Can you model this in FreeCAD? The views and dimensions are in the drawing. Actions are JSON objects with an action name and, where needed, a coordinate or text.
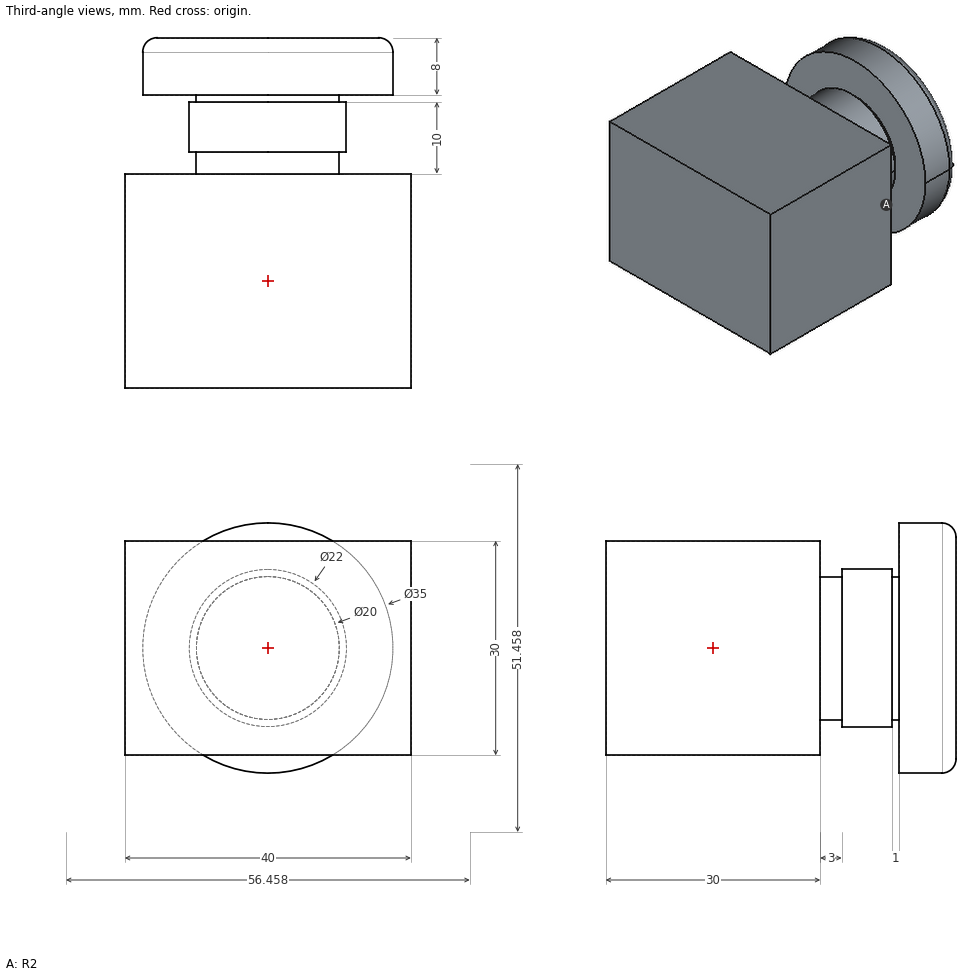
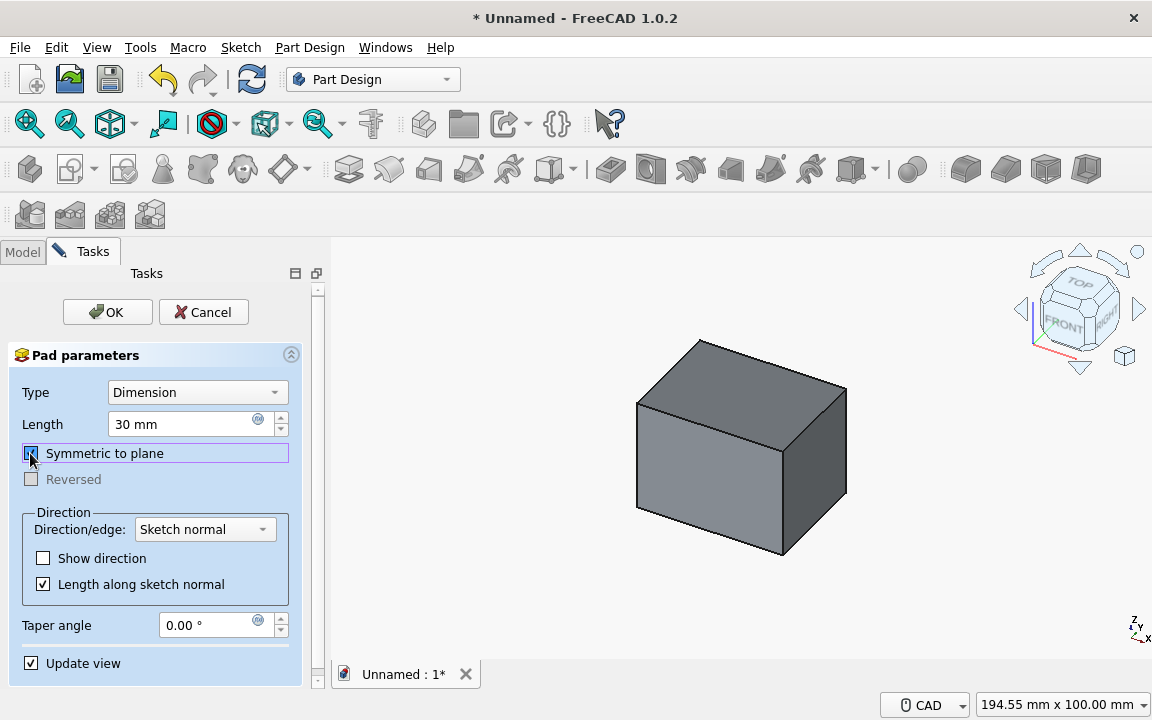
{"action": "left_click", "coordinate": [108, 312]}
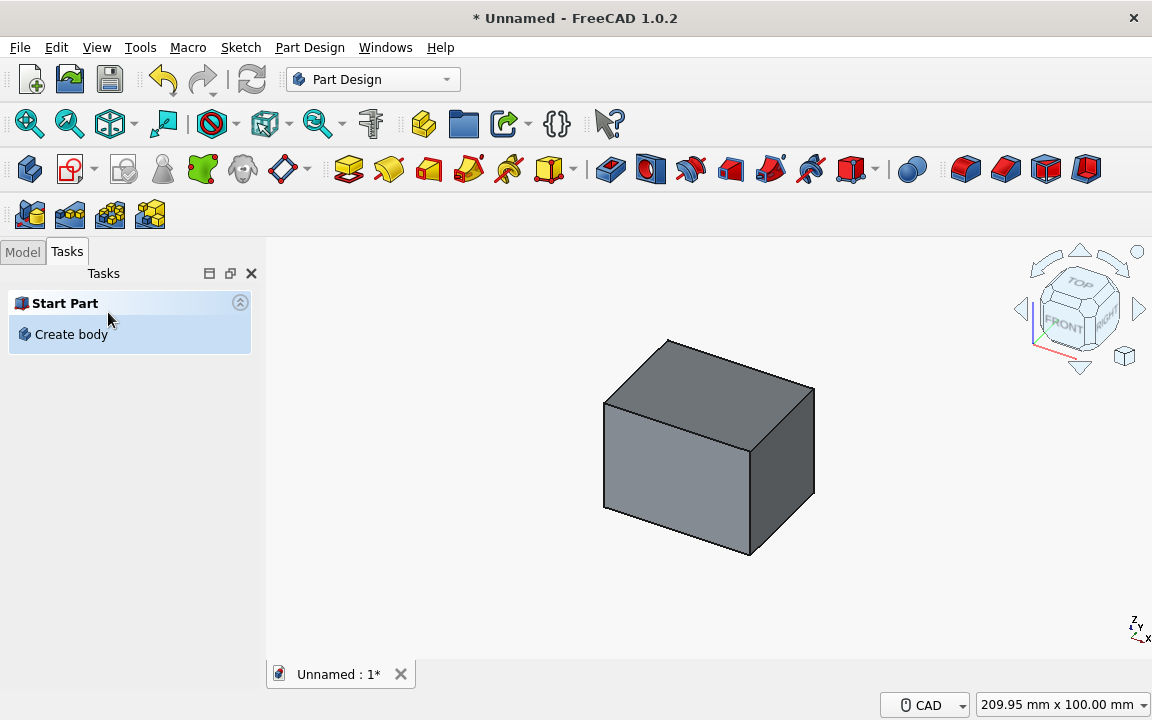
{"action": "key", "text": "4"}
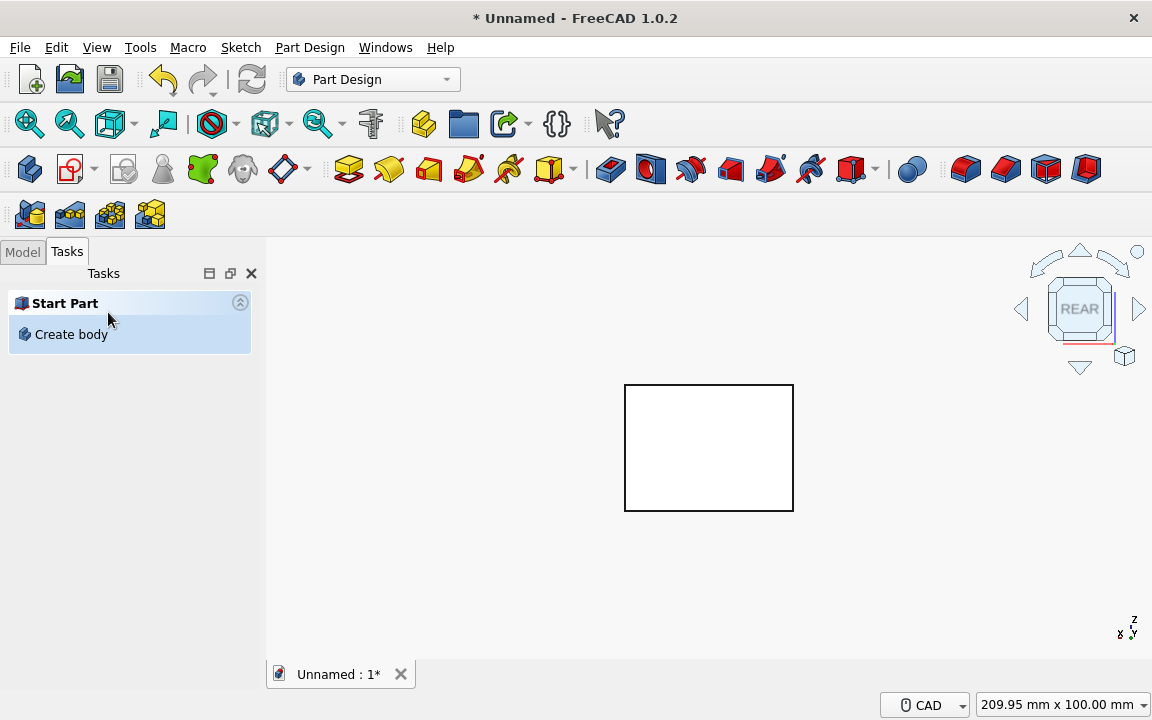
{"action": "left_click", "coordinate": [30, 124]}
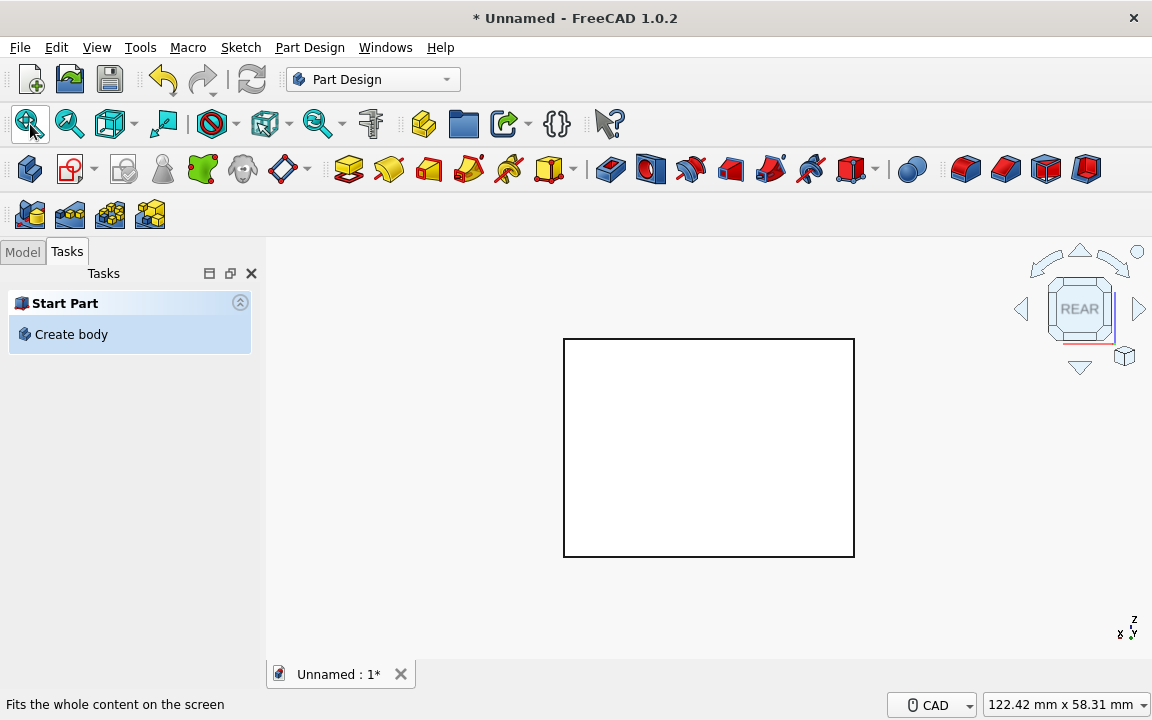
{"action": "left_click", "coordinate": [709, 447]}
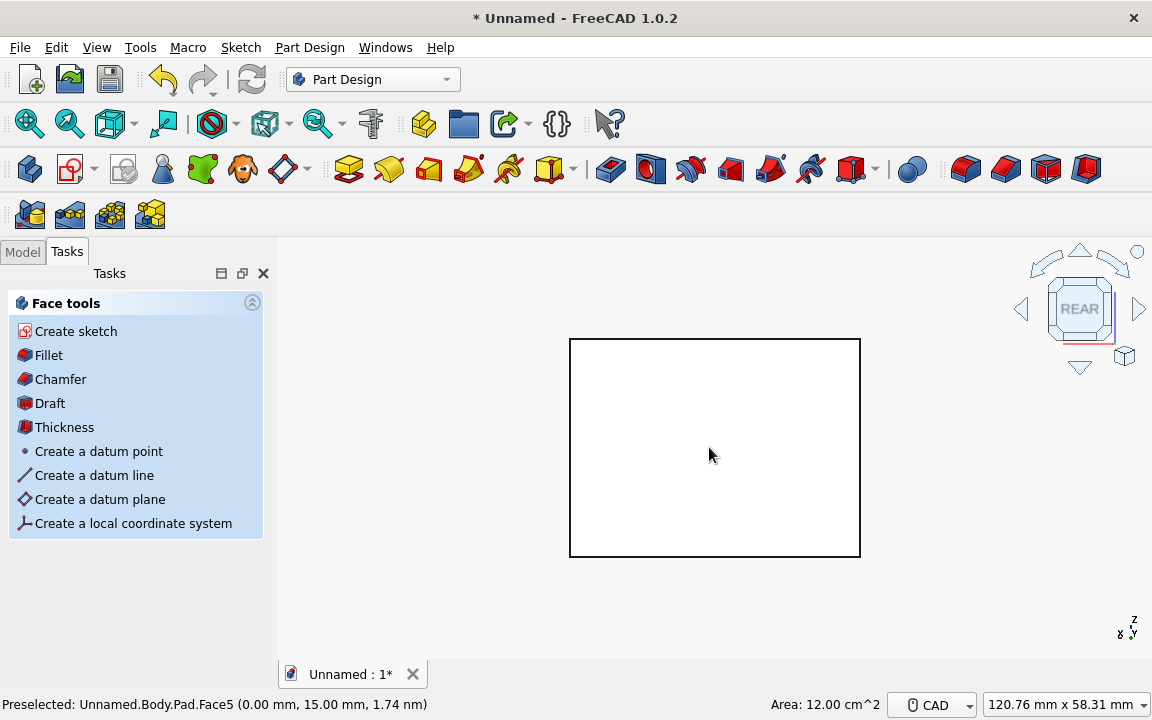
{"action": "left_click", "coordinate": [70, 170]}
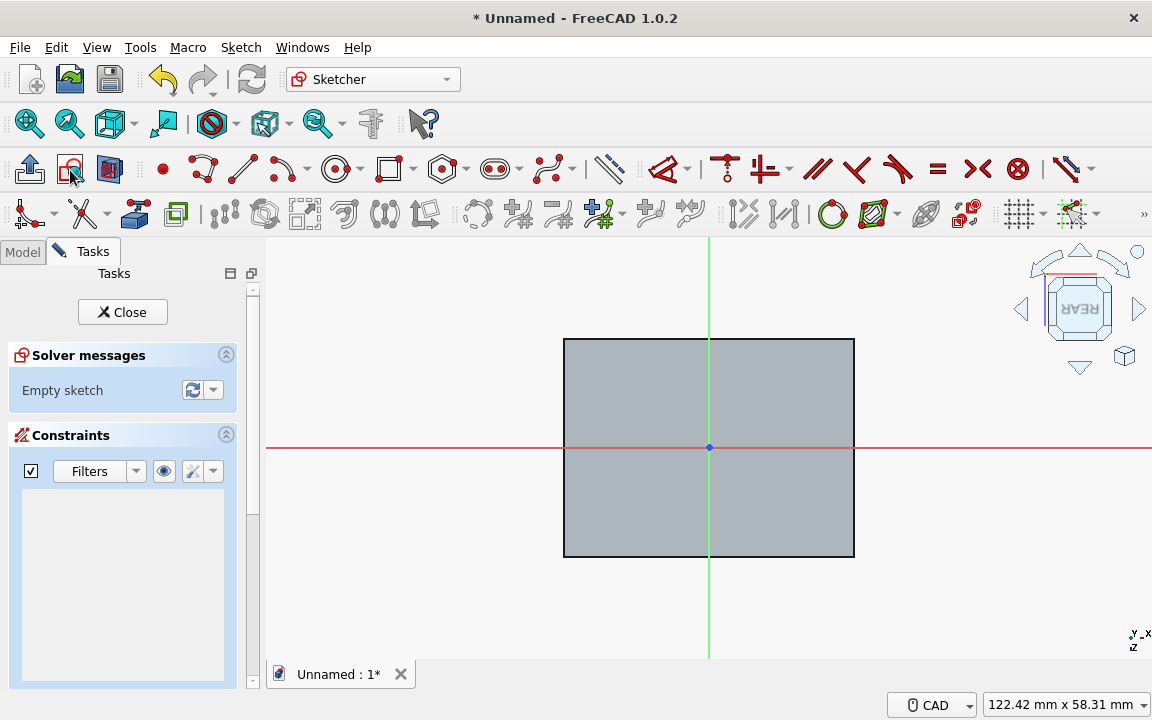
{"action": "scroll", "coordinate": [848, 448], "scroll_direction": "up", "scroll_amount": 2}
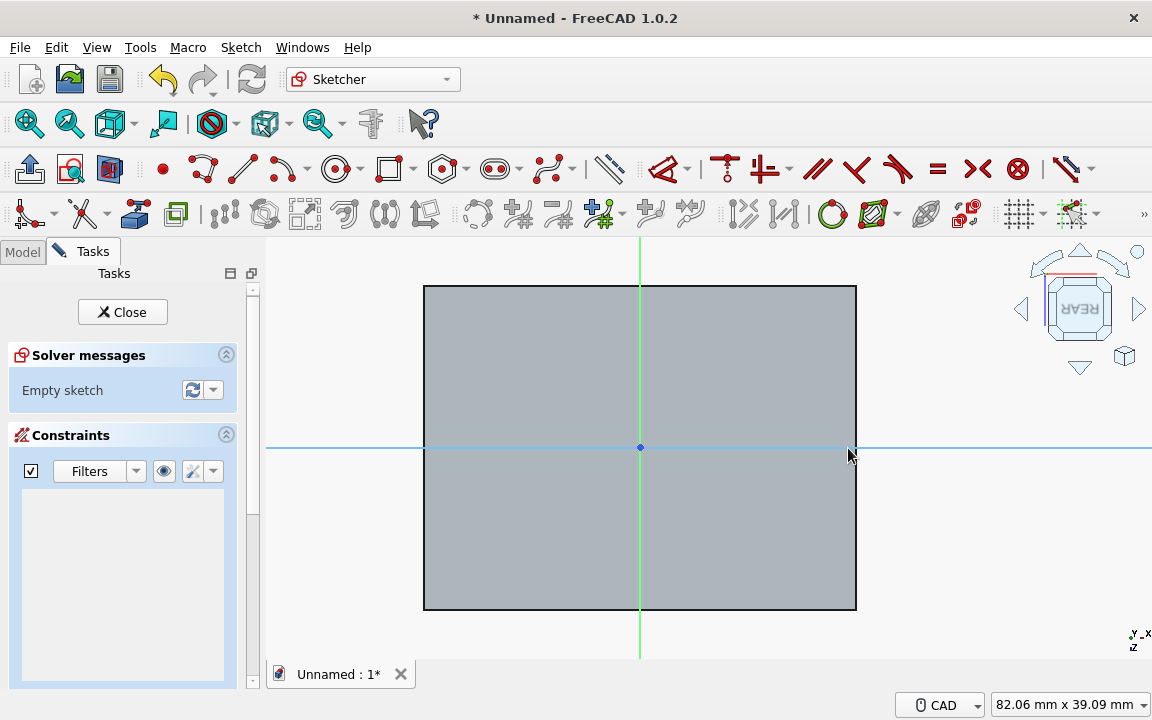
{"action": "left_click", "coordinate": [336, 170]}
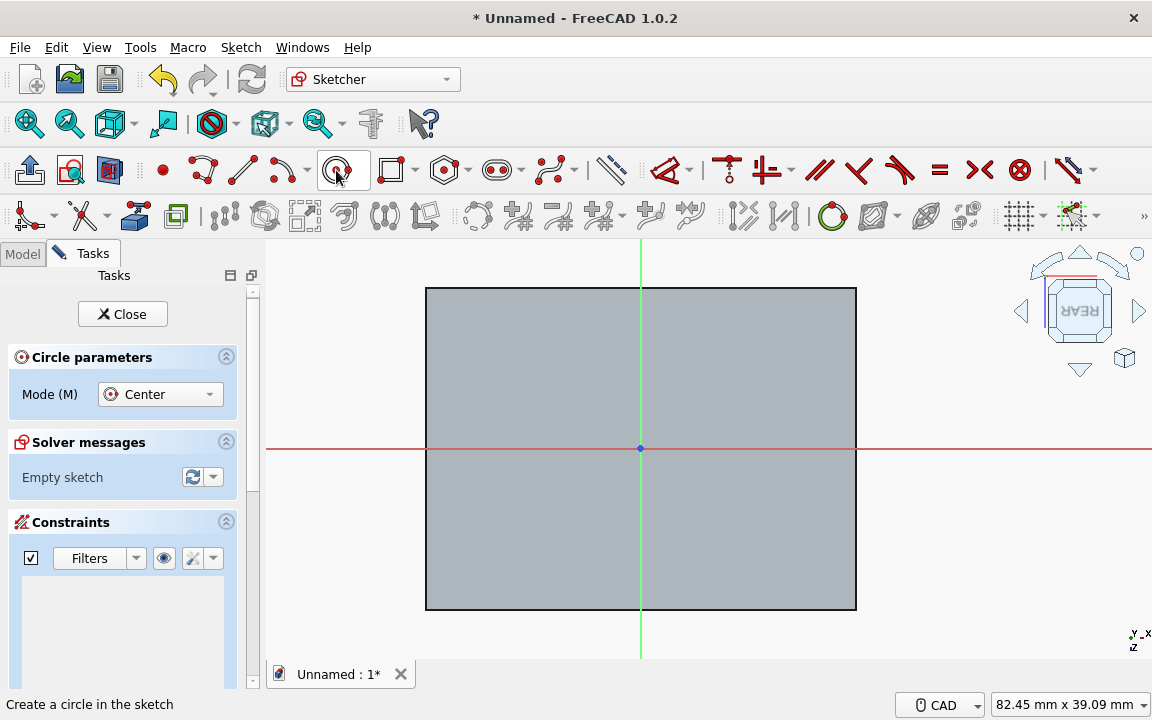
{"action": "left_click", "coordinate": [641, 449]}
{"action": "mouse_move", "coordinate": [724, 365]}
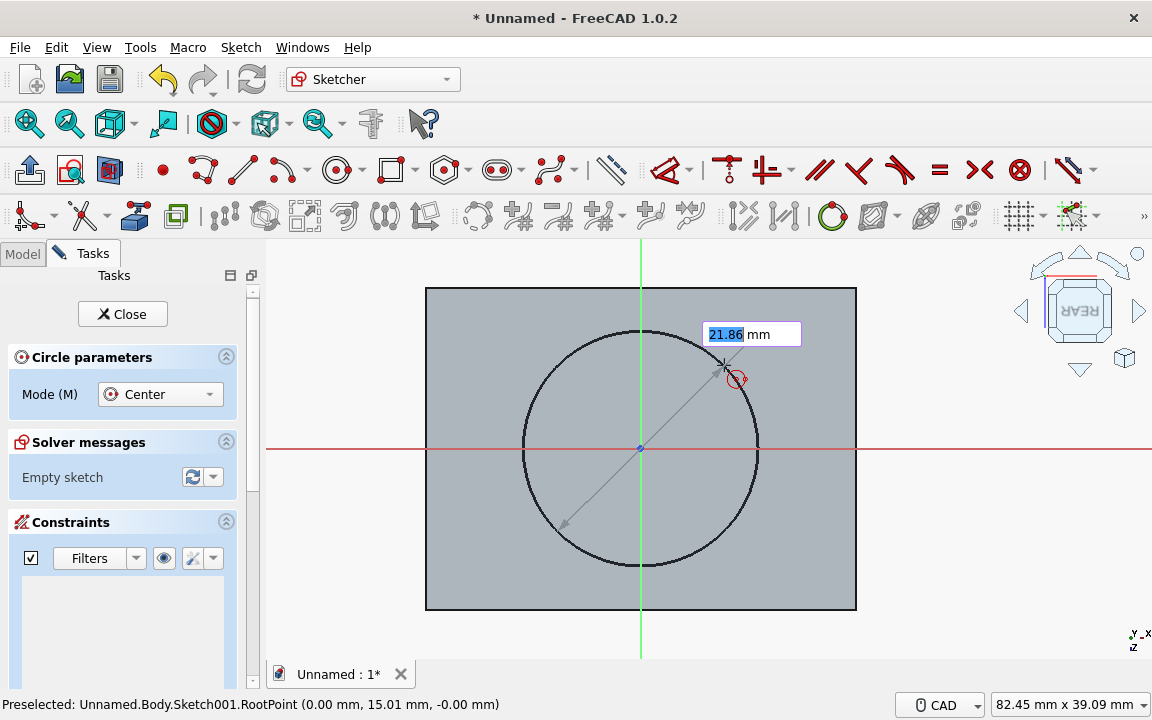
{"action": "type", "text": "22"}
{"action": "key", "text": "Return"}
{"action": "key", "text": "Escape"}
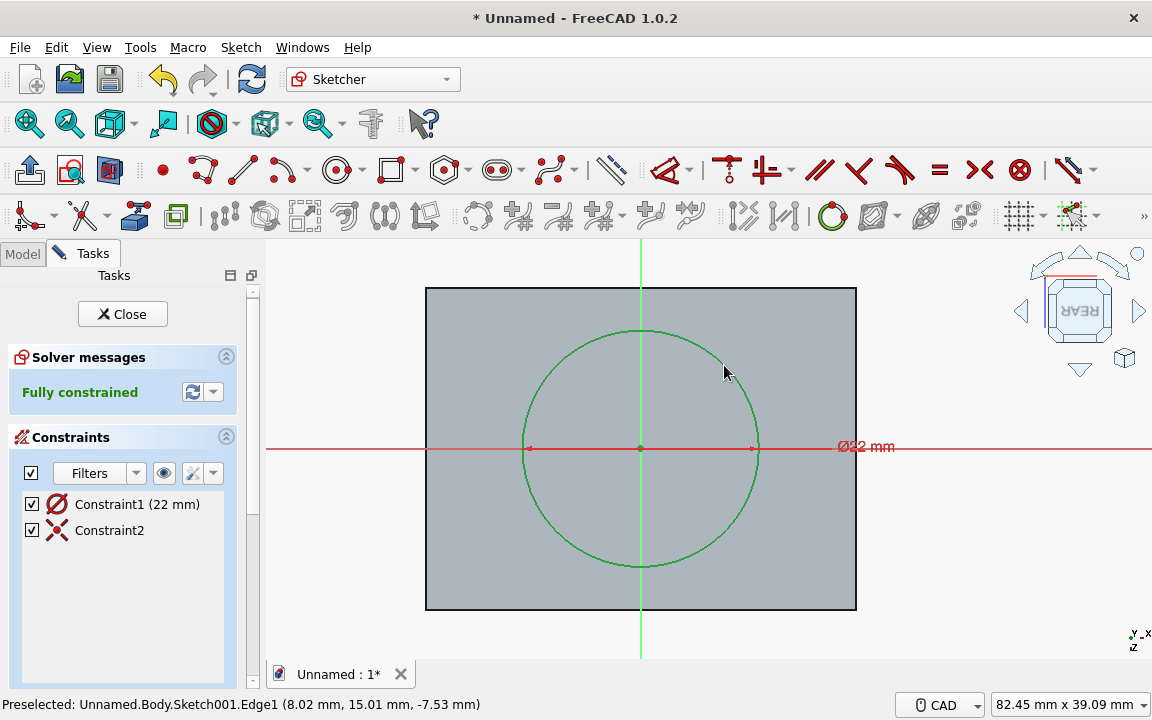
{"action": "left_click", "coordinate": [123, 314]}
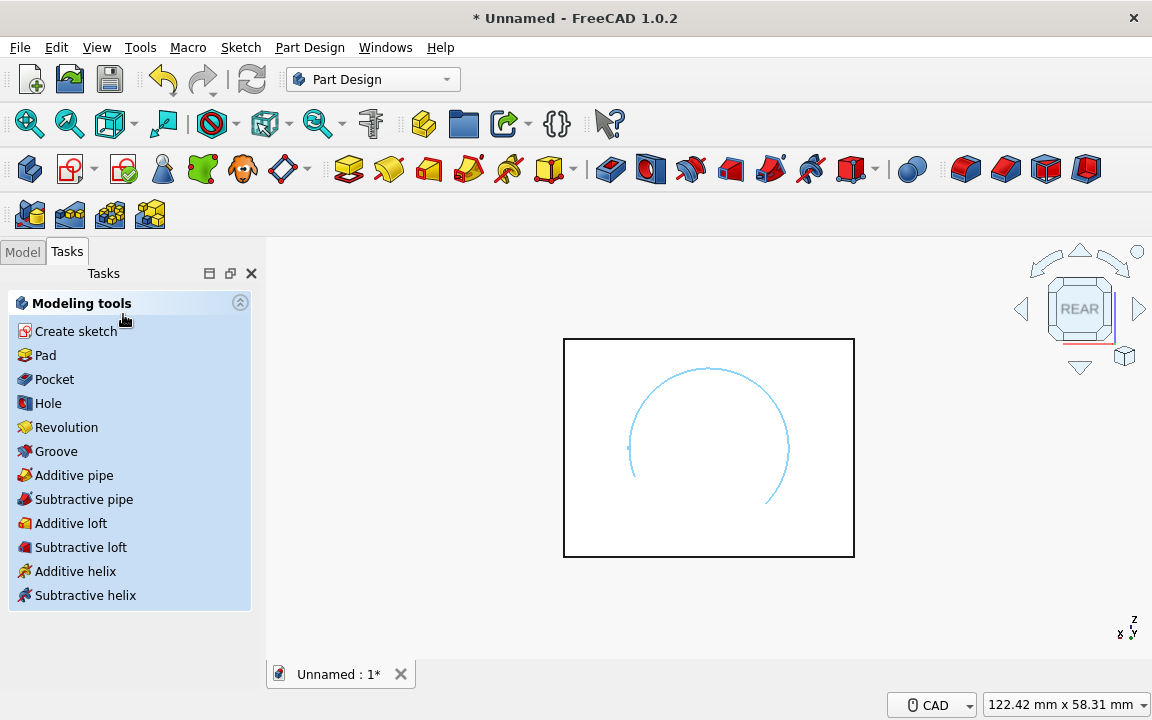
{"action": "left_click", "coordinate": [350, 170]}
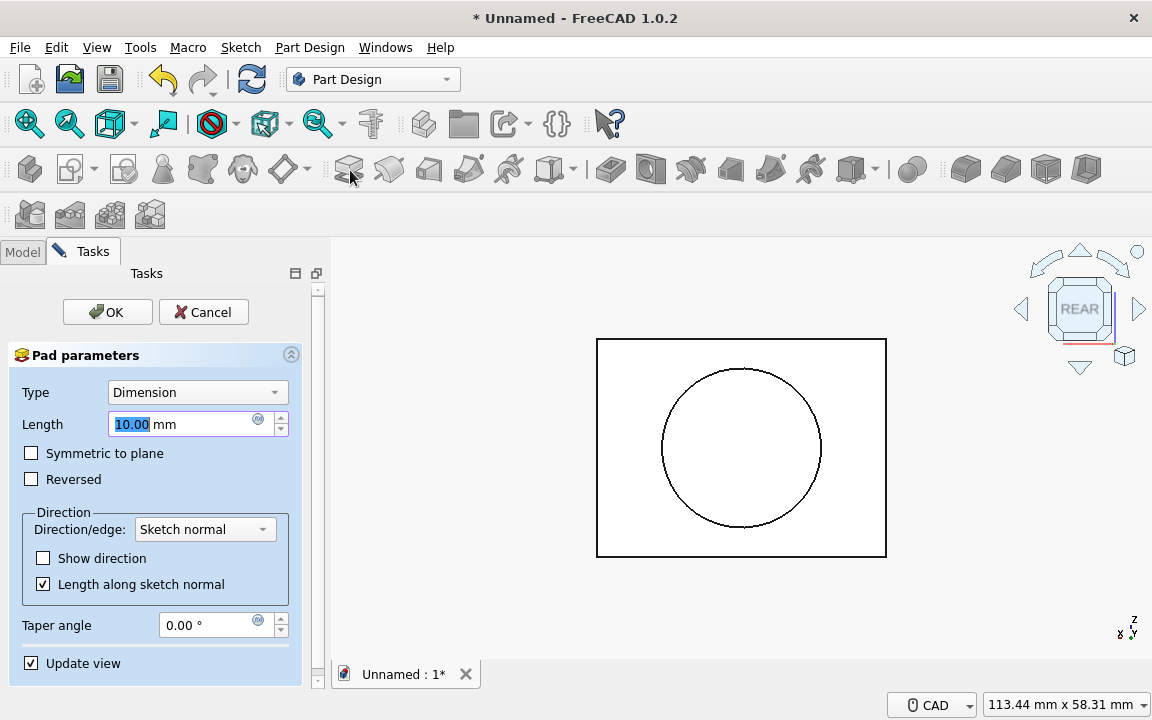
{"action": "type", "text": "10"}
{"action": "key", "text": "Tab"}